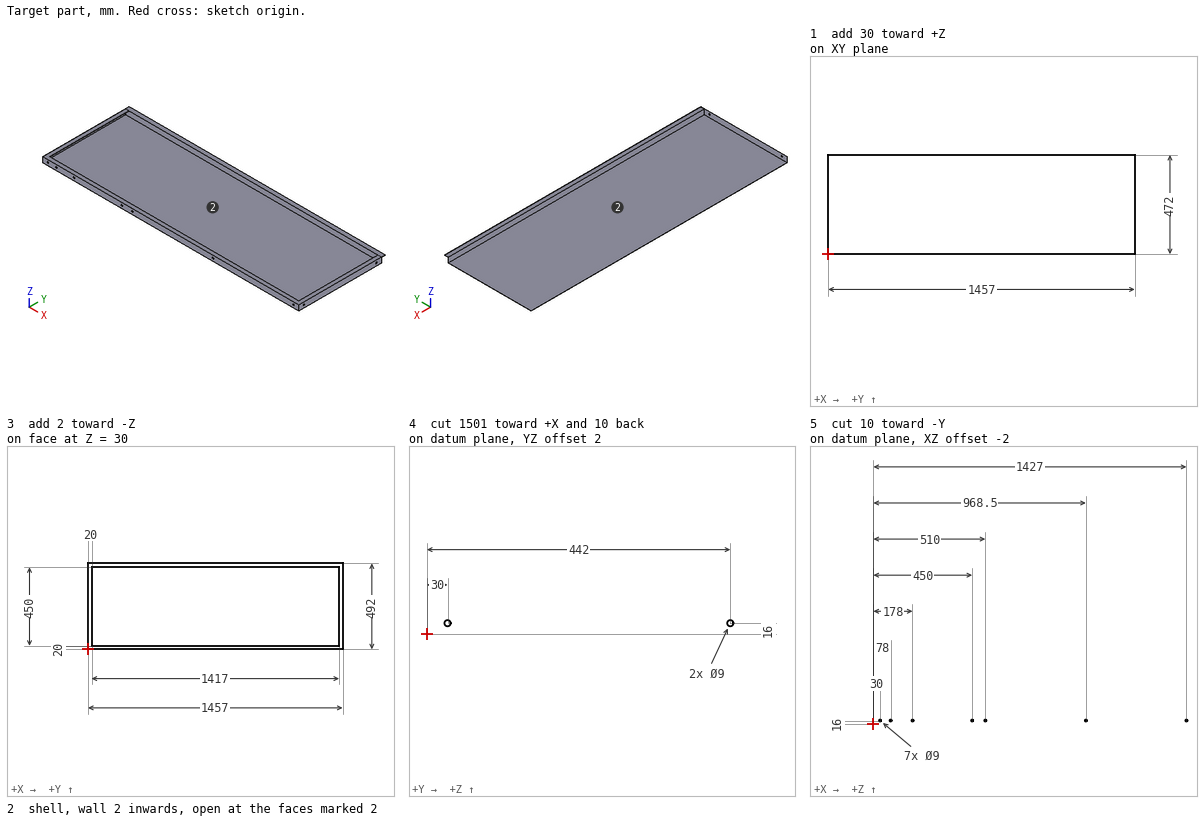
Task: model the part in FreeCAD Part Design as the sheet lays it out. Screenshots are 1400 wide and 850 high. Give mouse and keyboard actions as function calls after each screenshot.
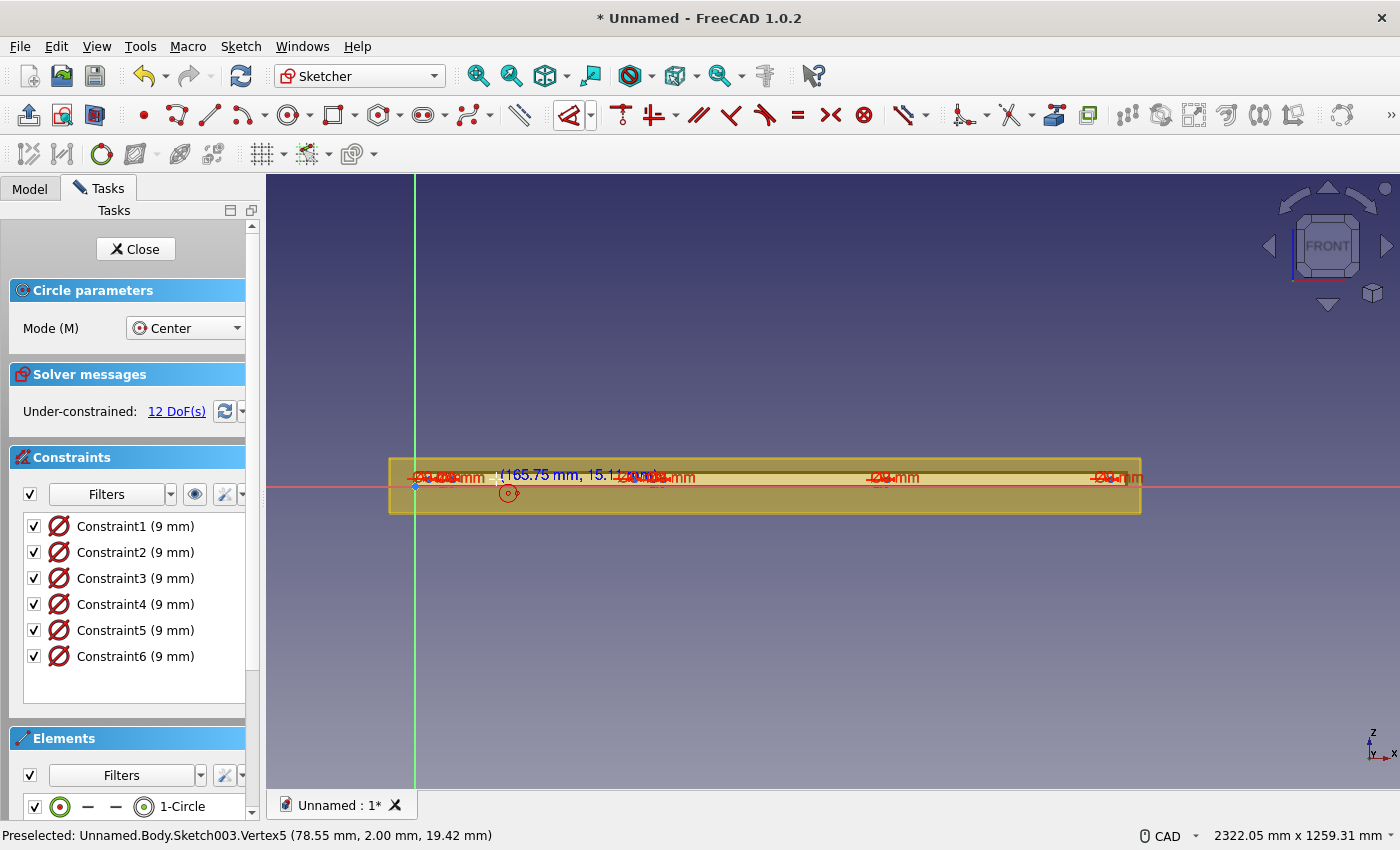
scroll(502, 479, up, 4)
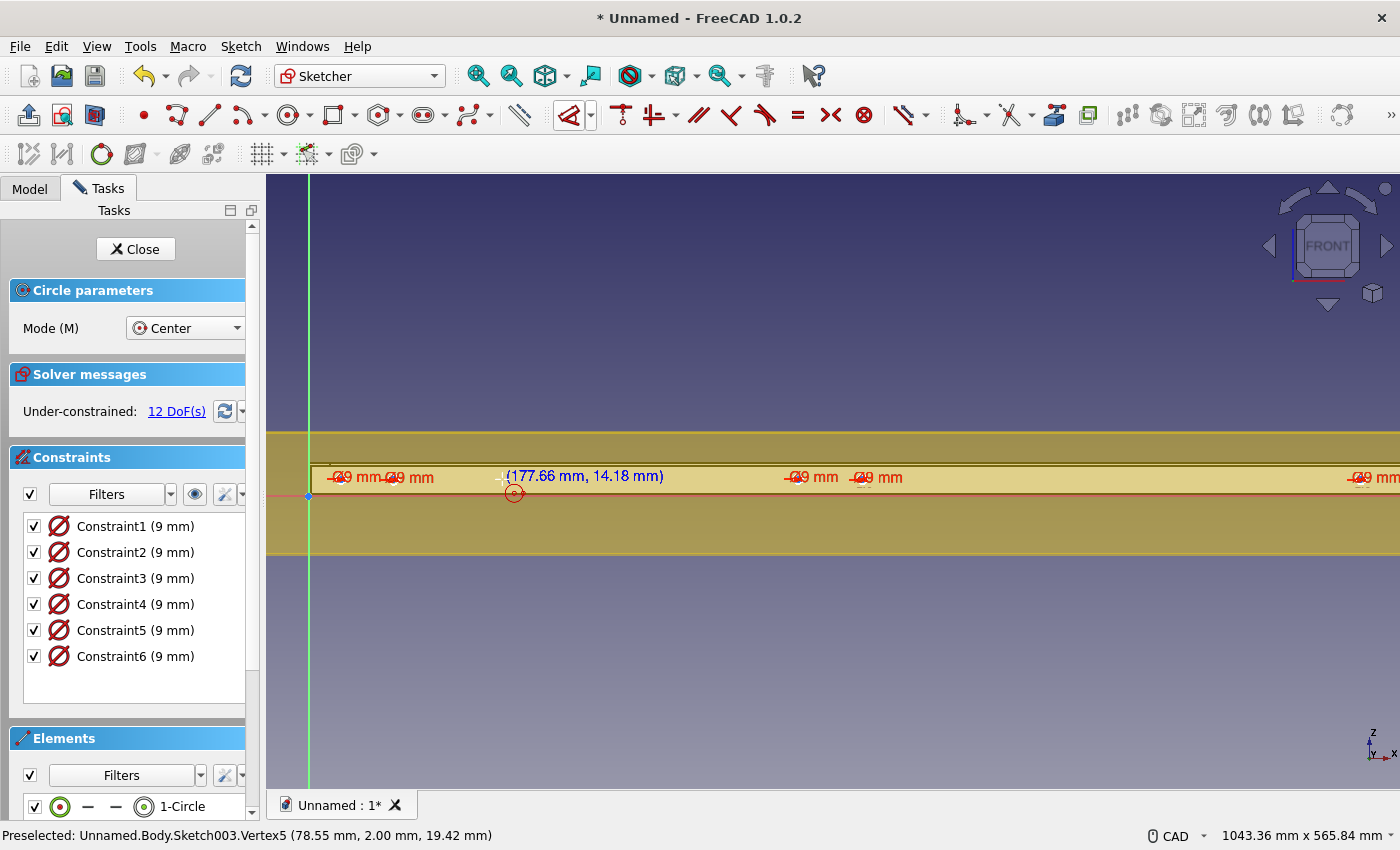
click(502, 479)
move(506, 475)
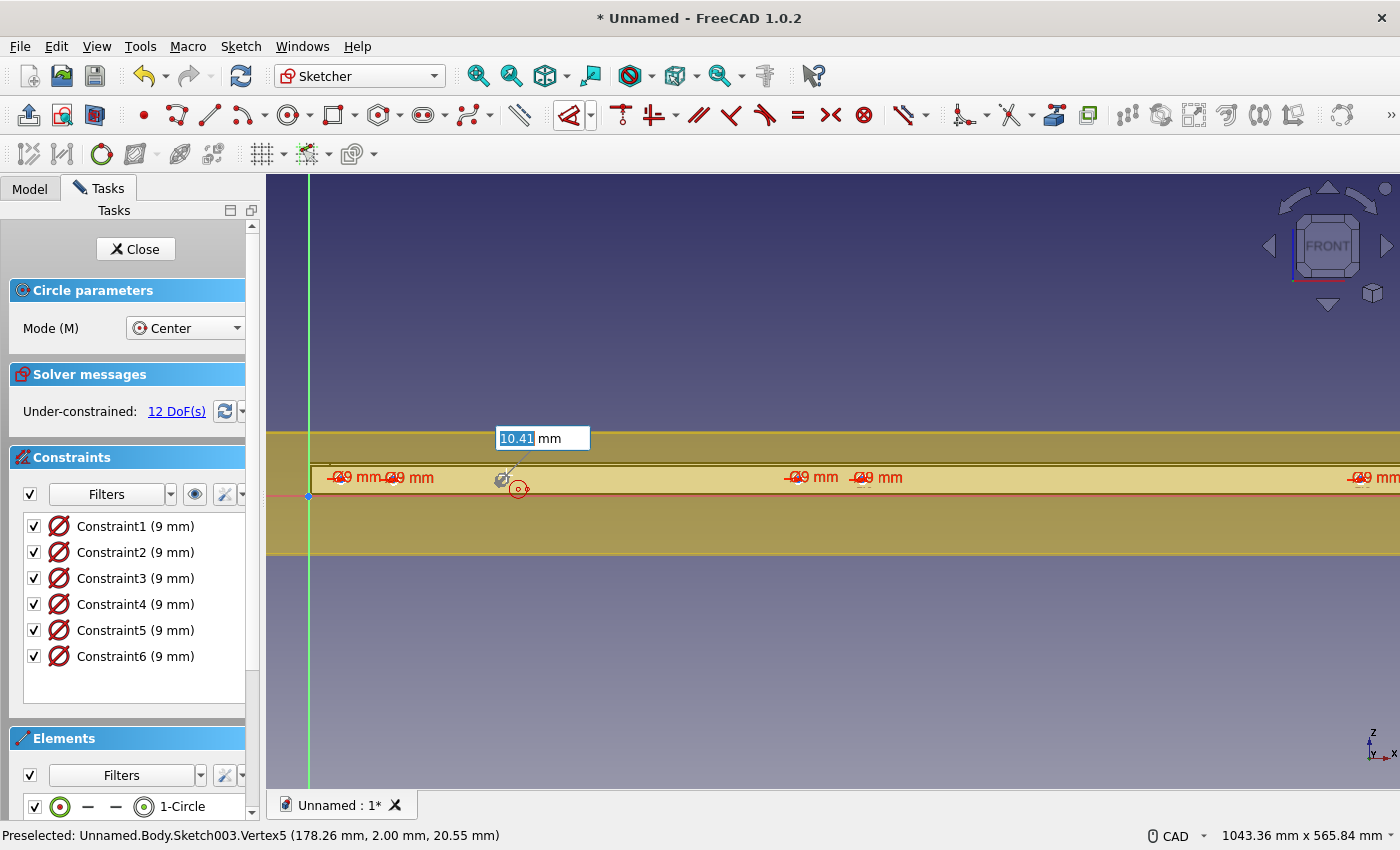
text(9)
key(Return)
key(Escape)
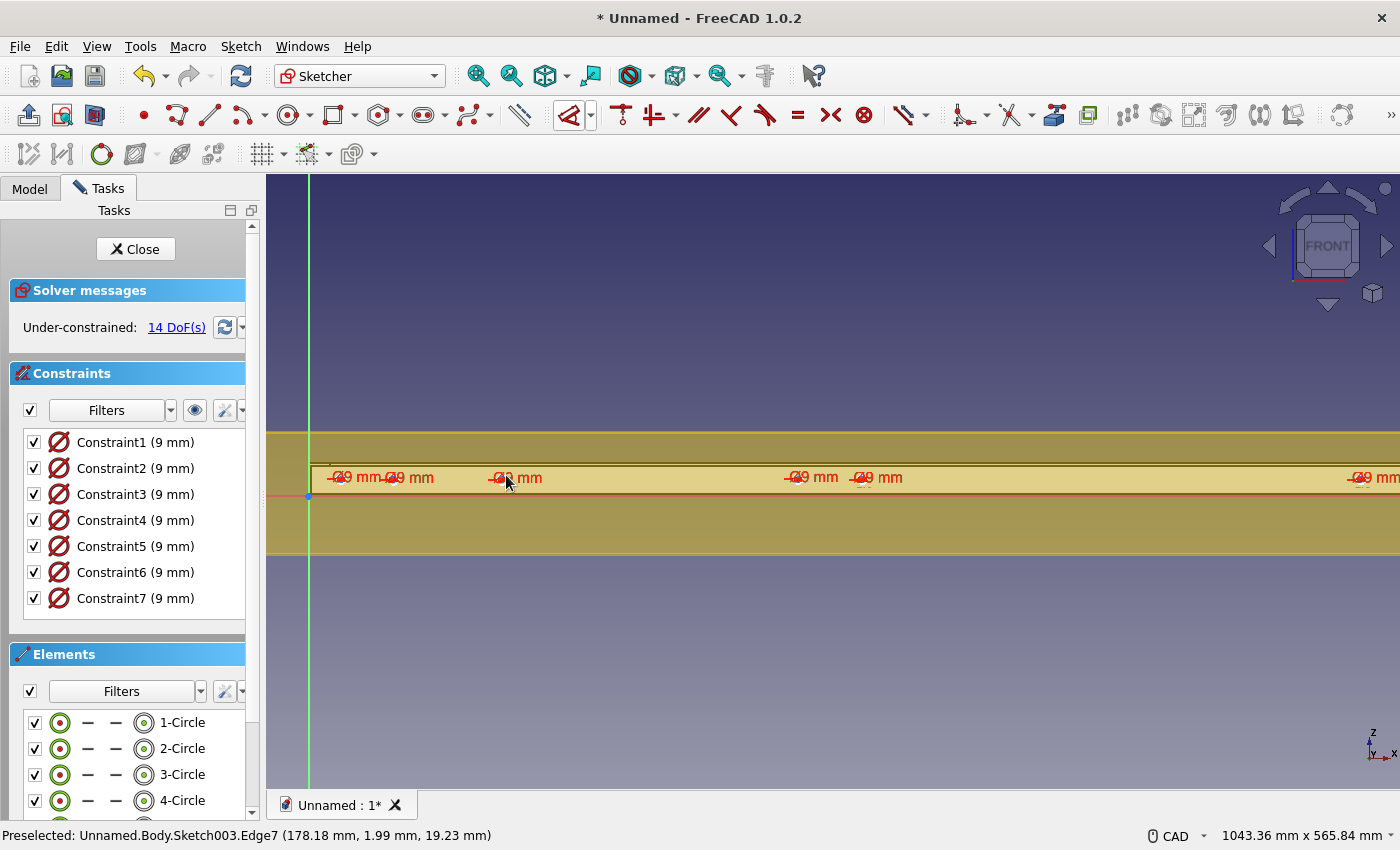
click(341, 479)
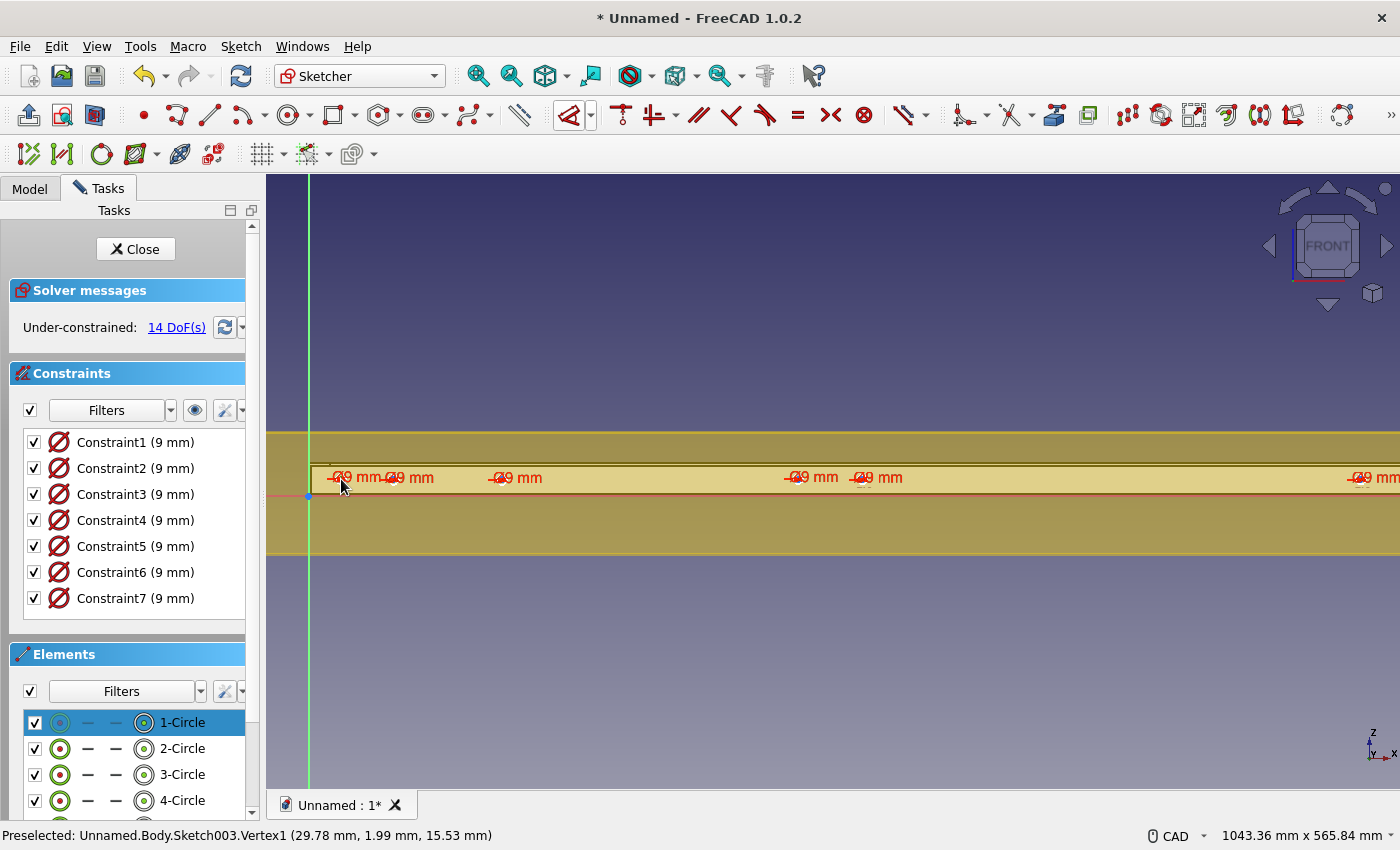
click(798, 479)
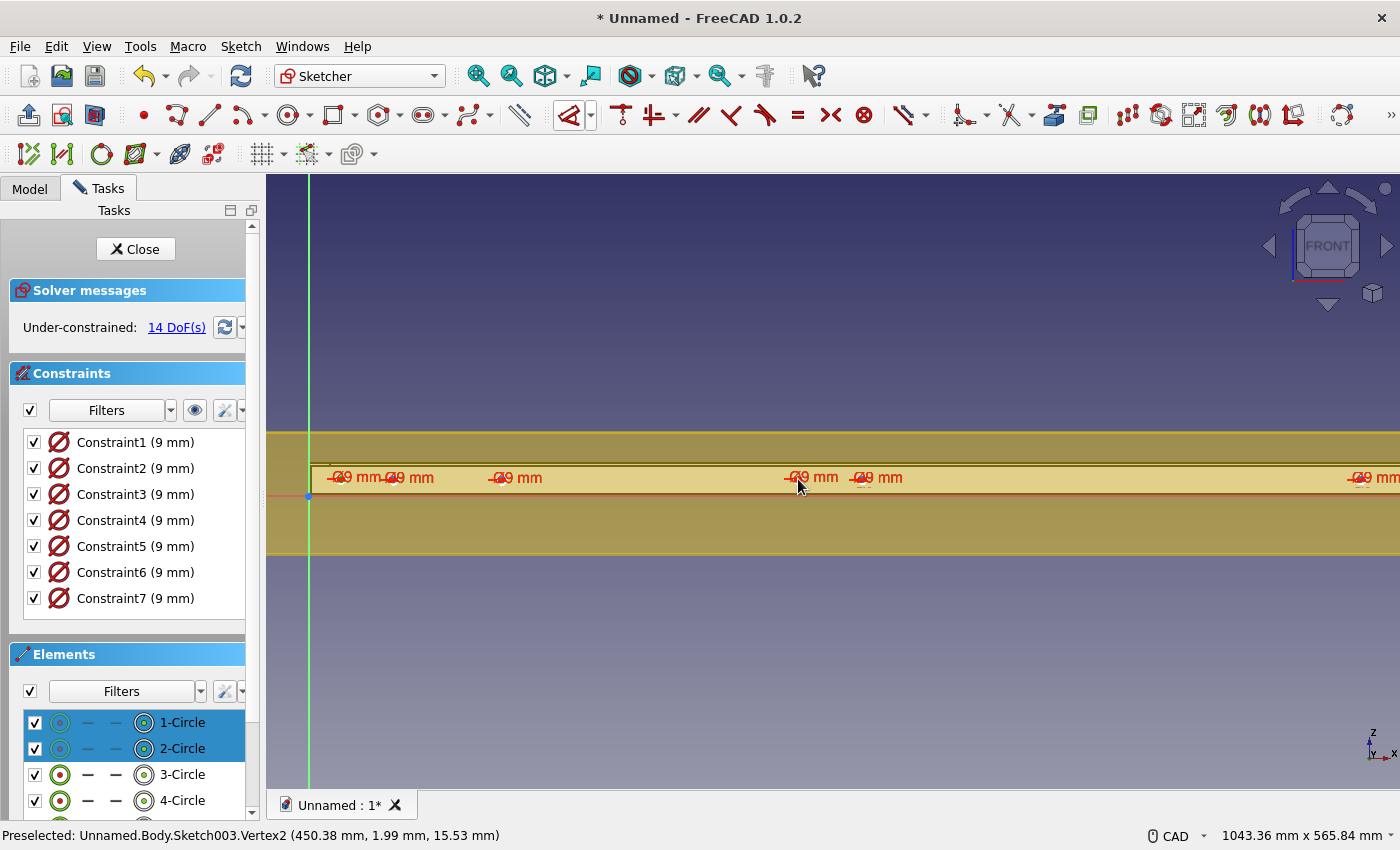
key(h)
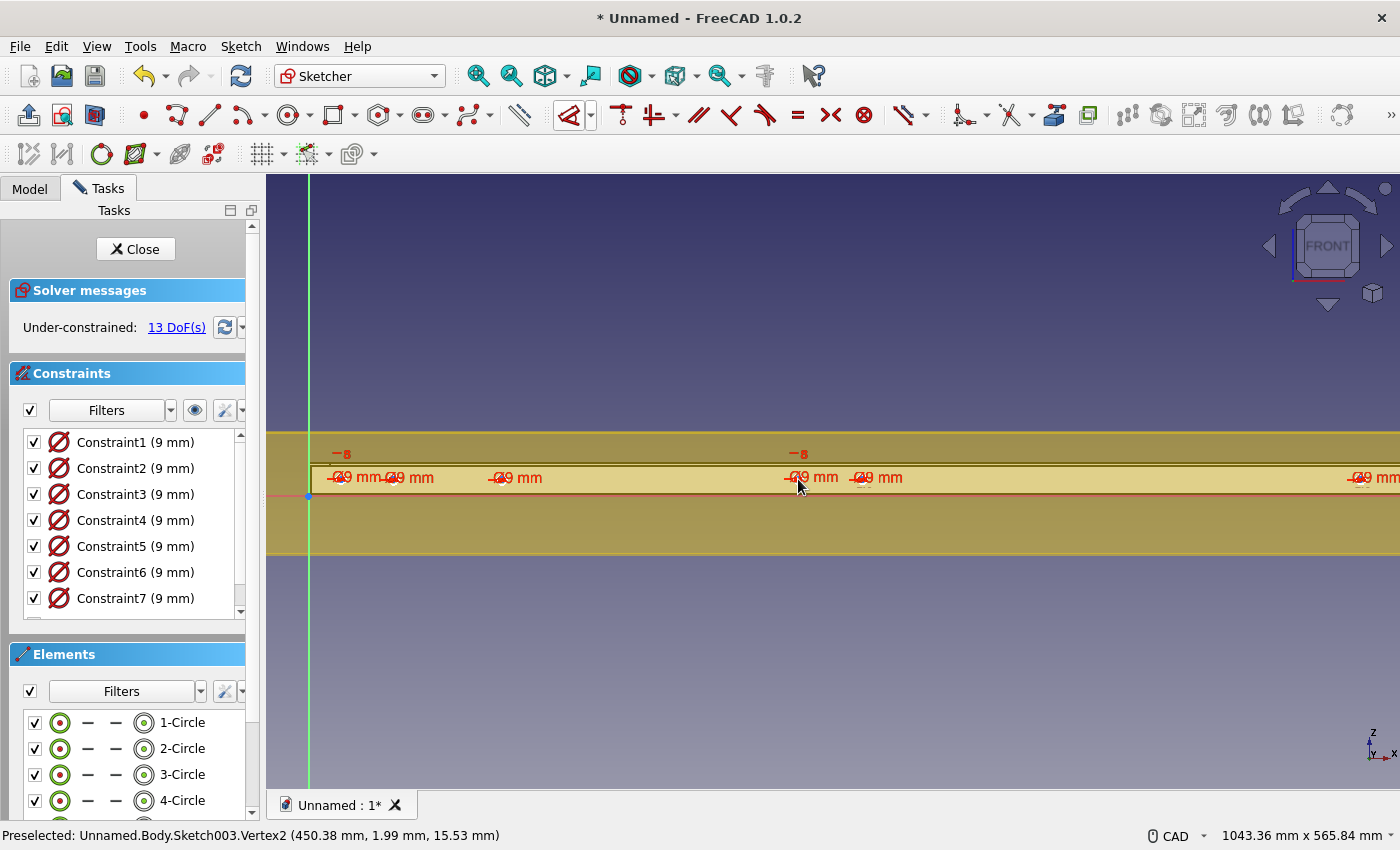
click(798, 479)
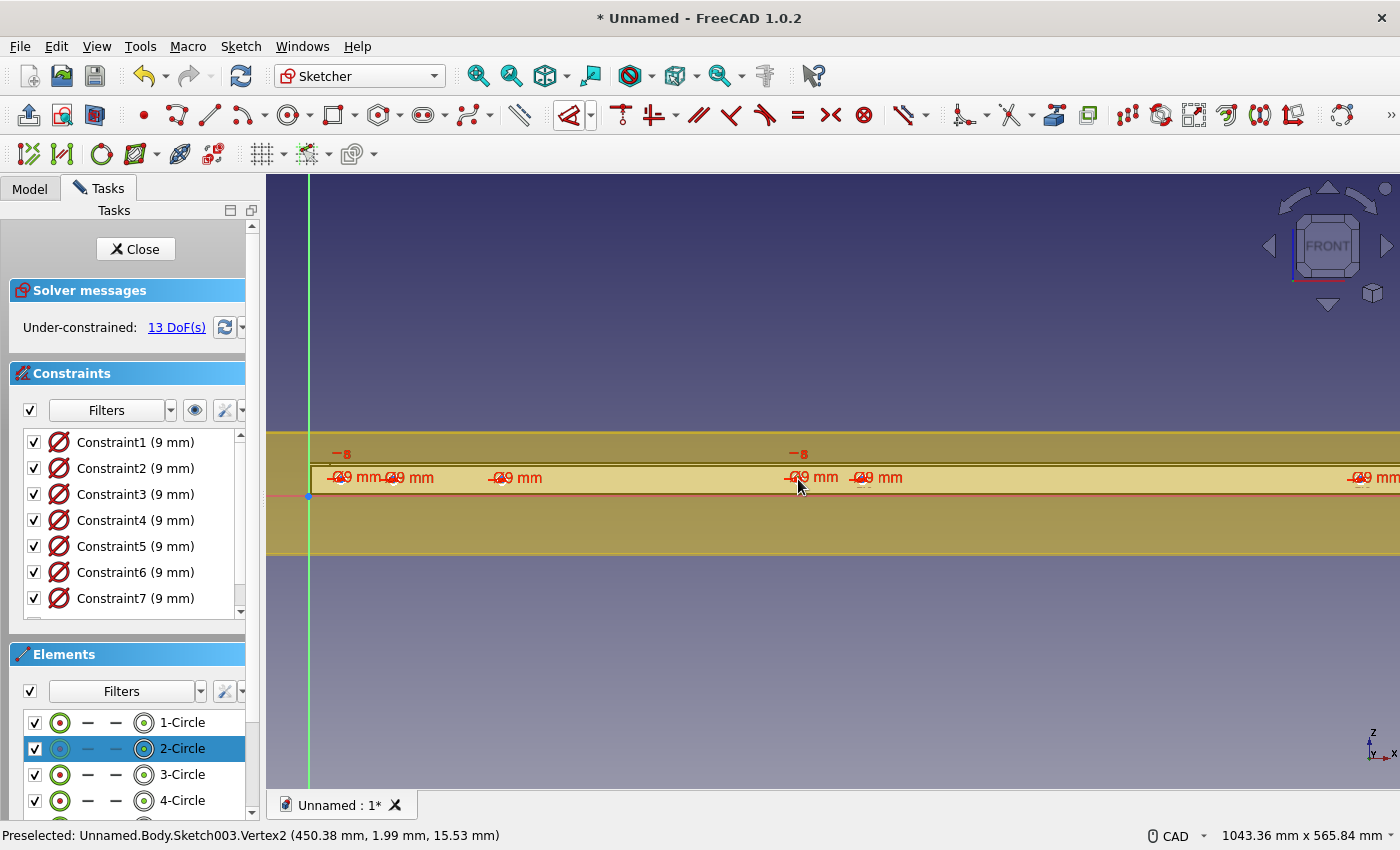
scroll(502, 479, down, 4)